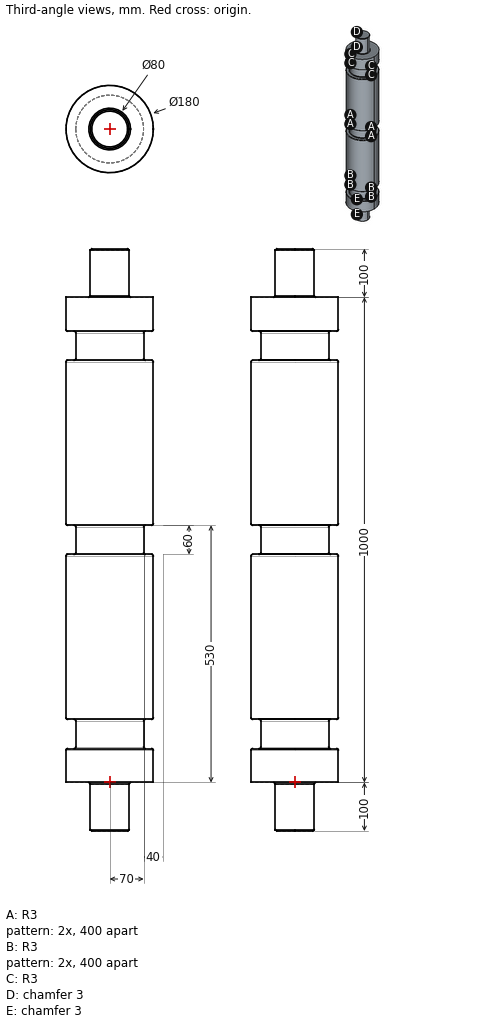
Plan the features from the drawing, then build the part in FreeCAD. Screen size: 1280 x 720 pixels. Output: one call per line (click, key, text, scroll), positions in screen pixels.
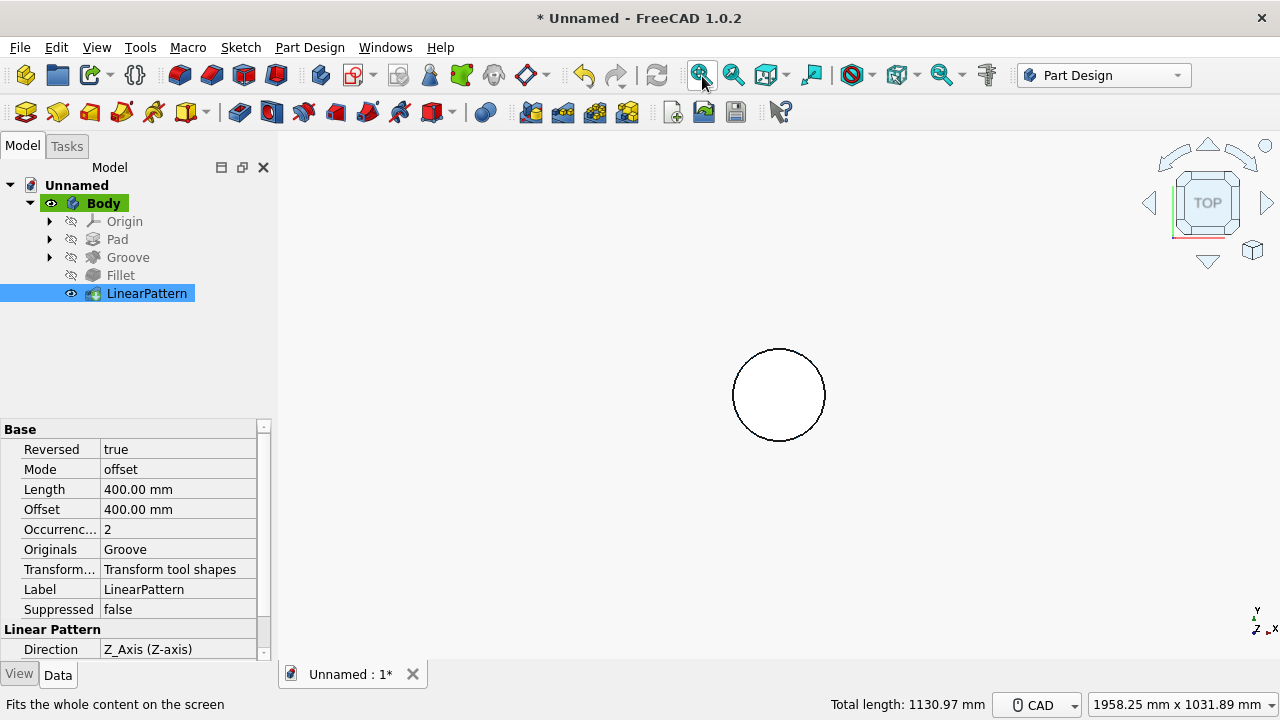
key(0)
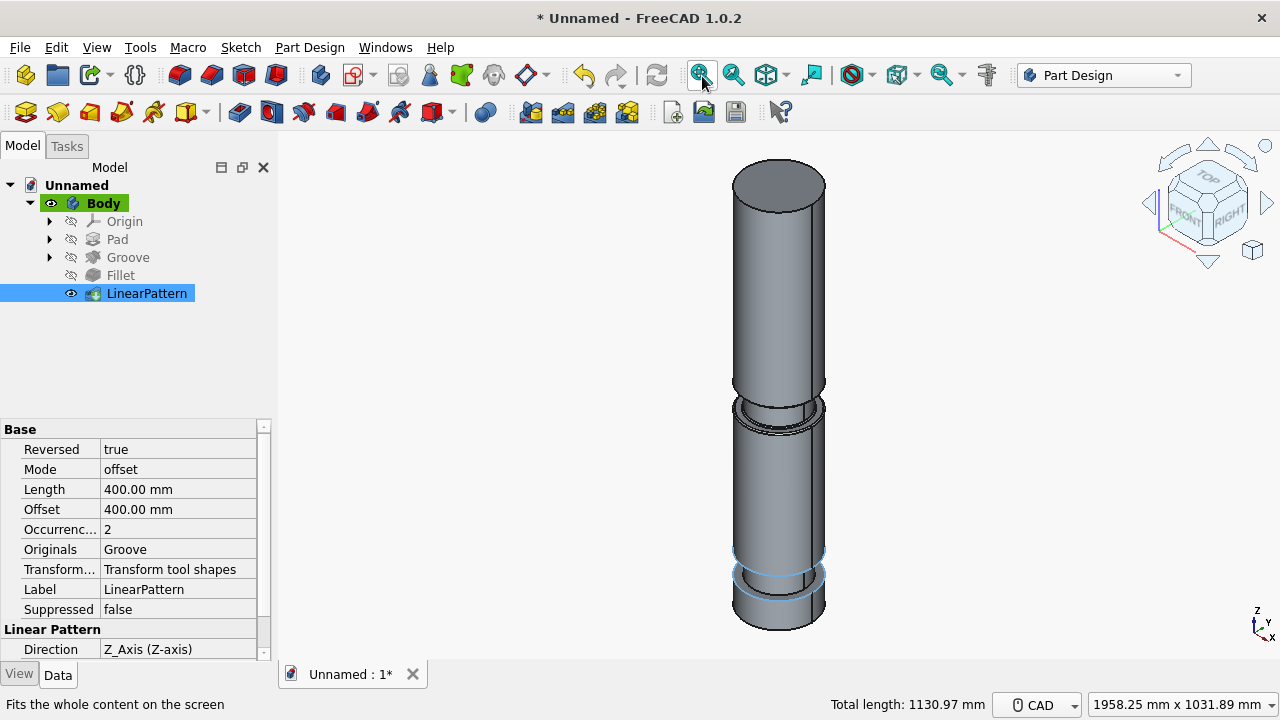
key(1)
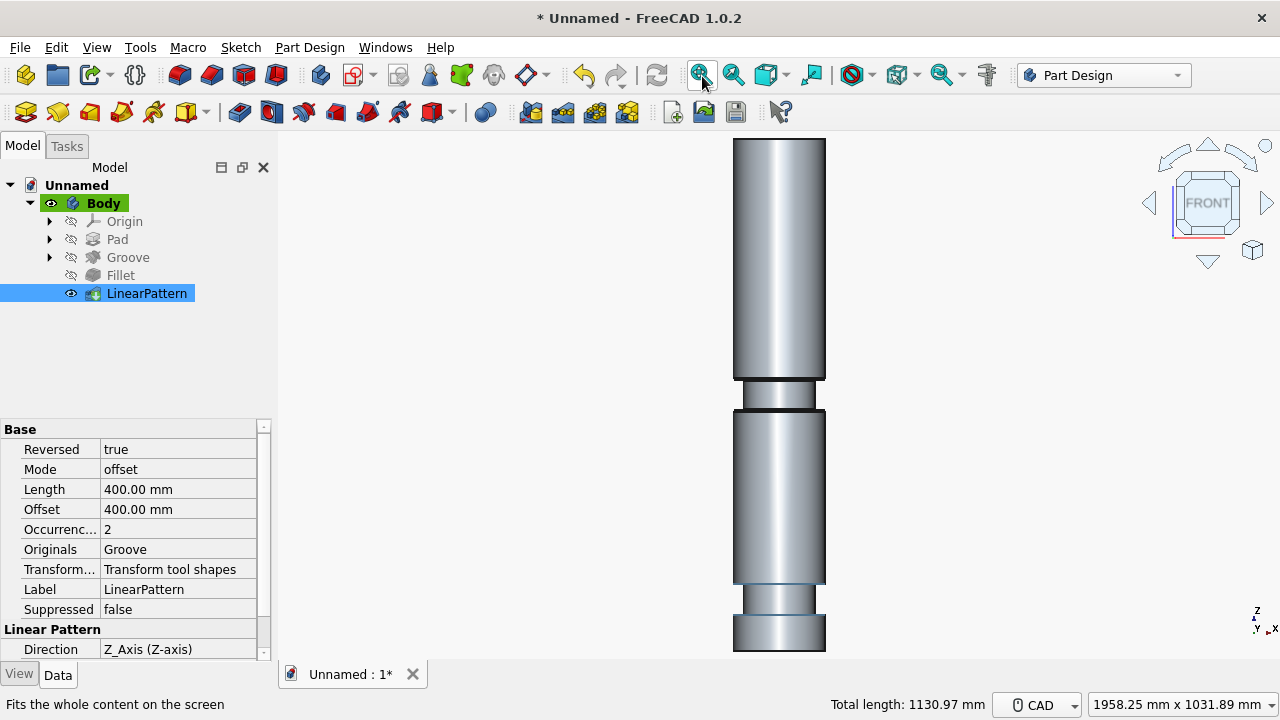
key(3)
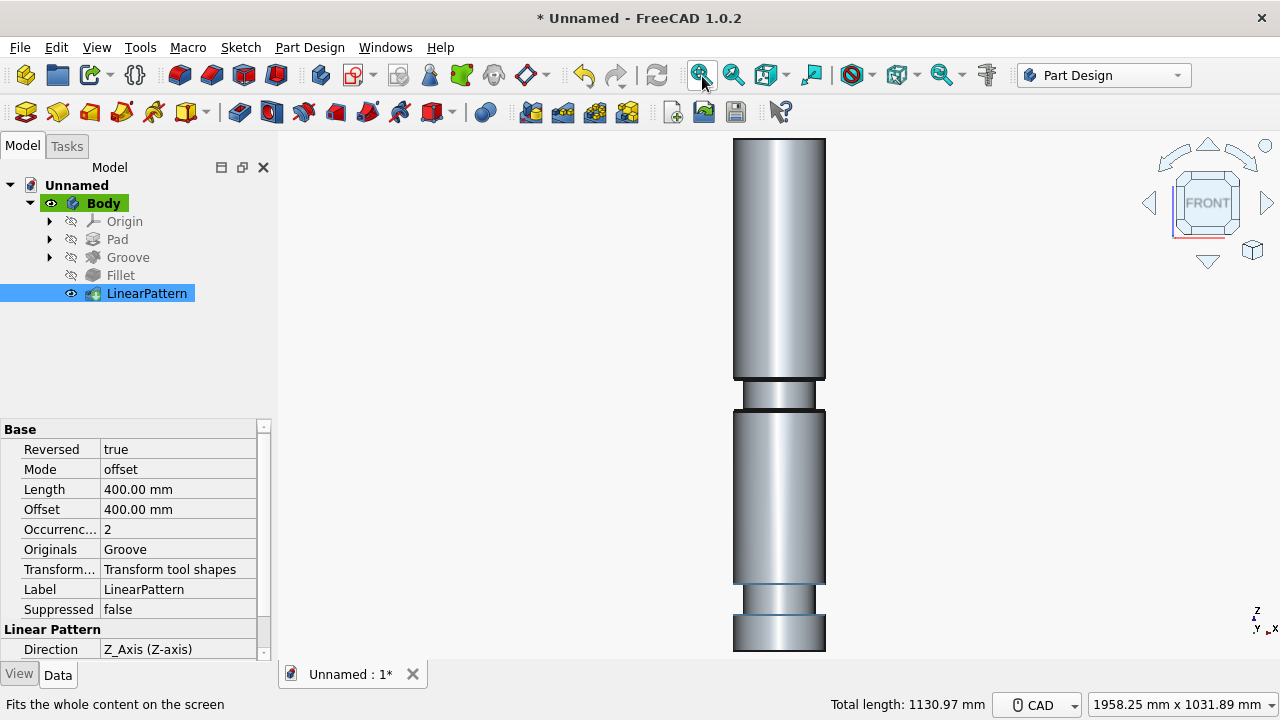
key(5)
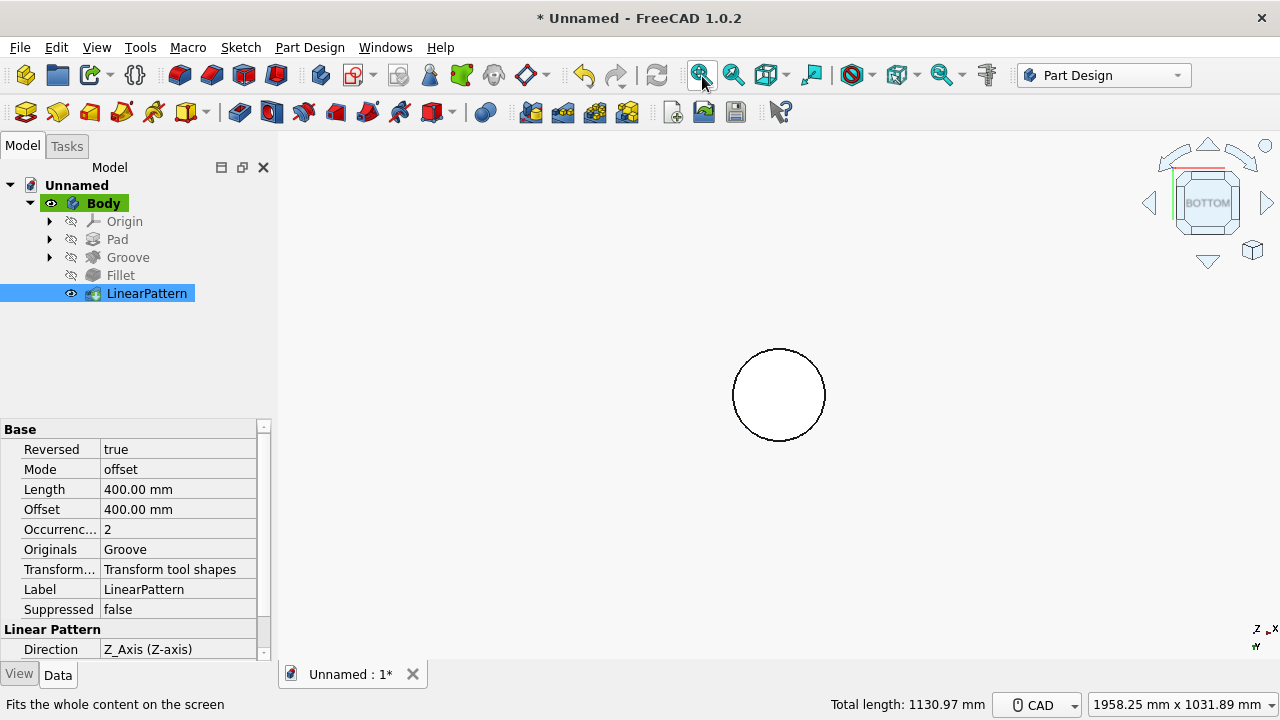
click(702, 76)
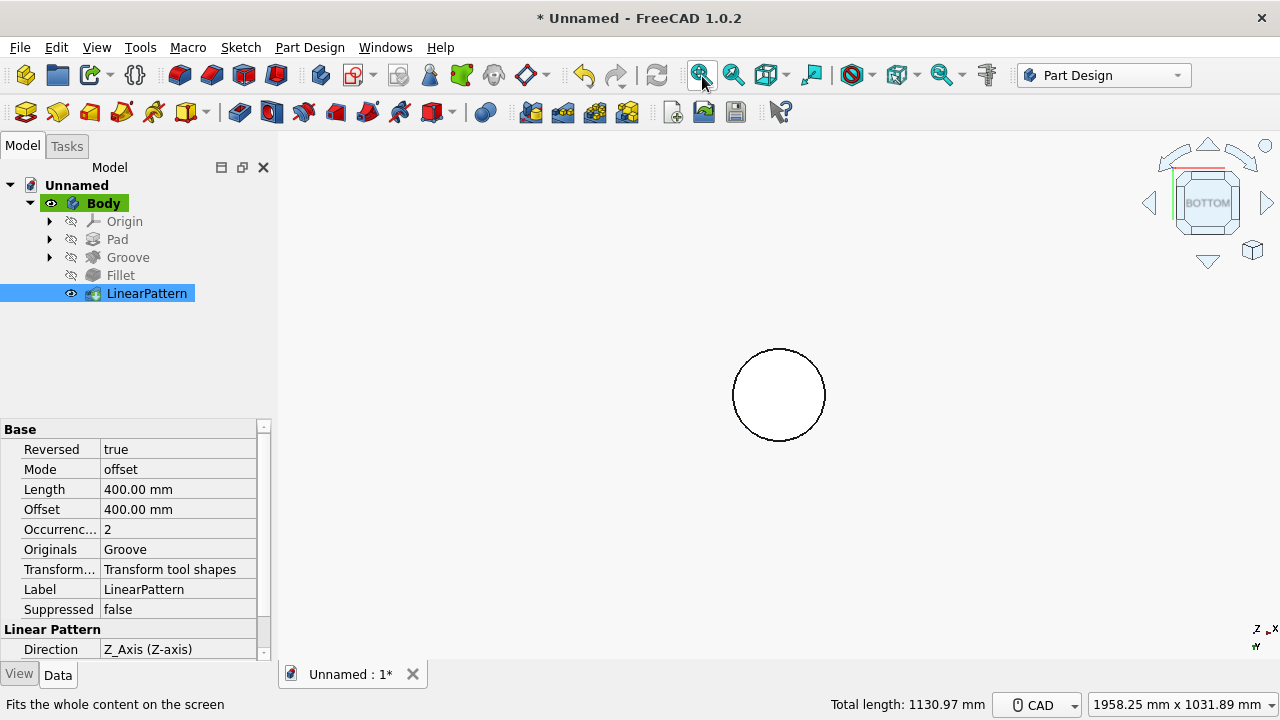
key(4)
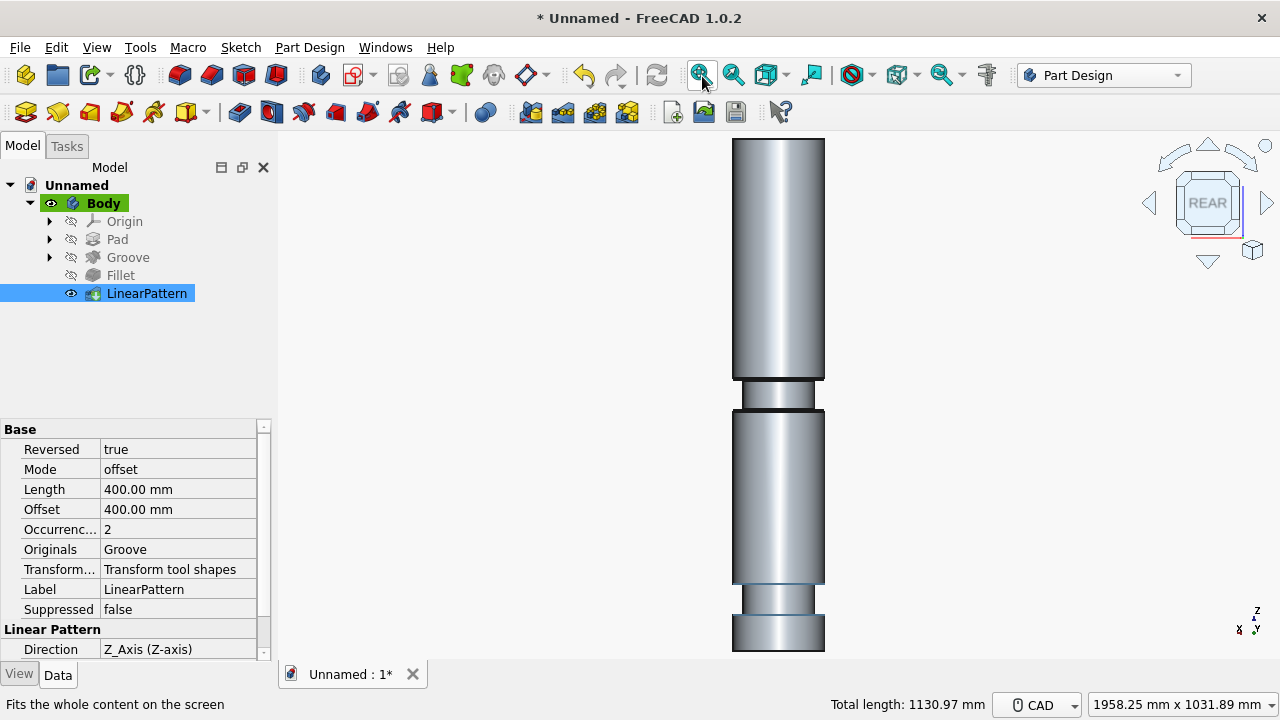
key(6)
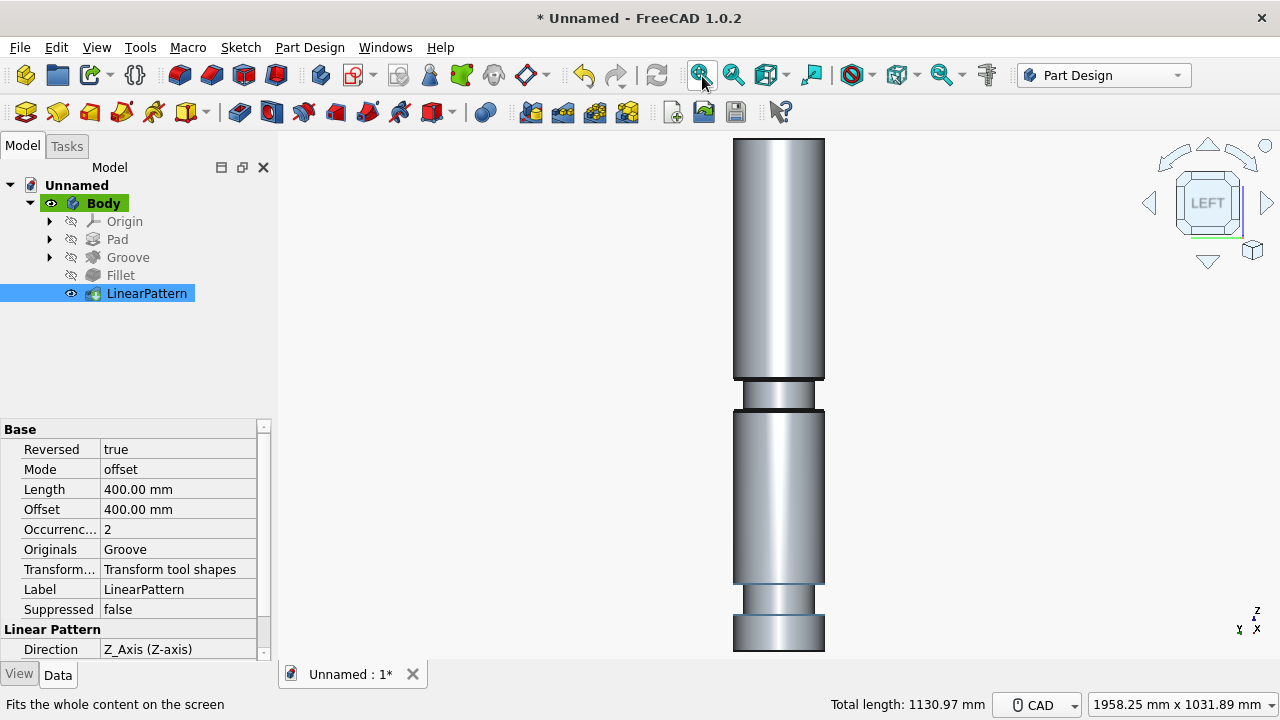
key(v)
key(3)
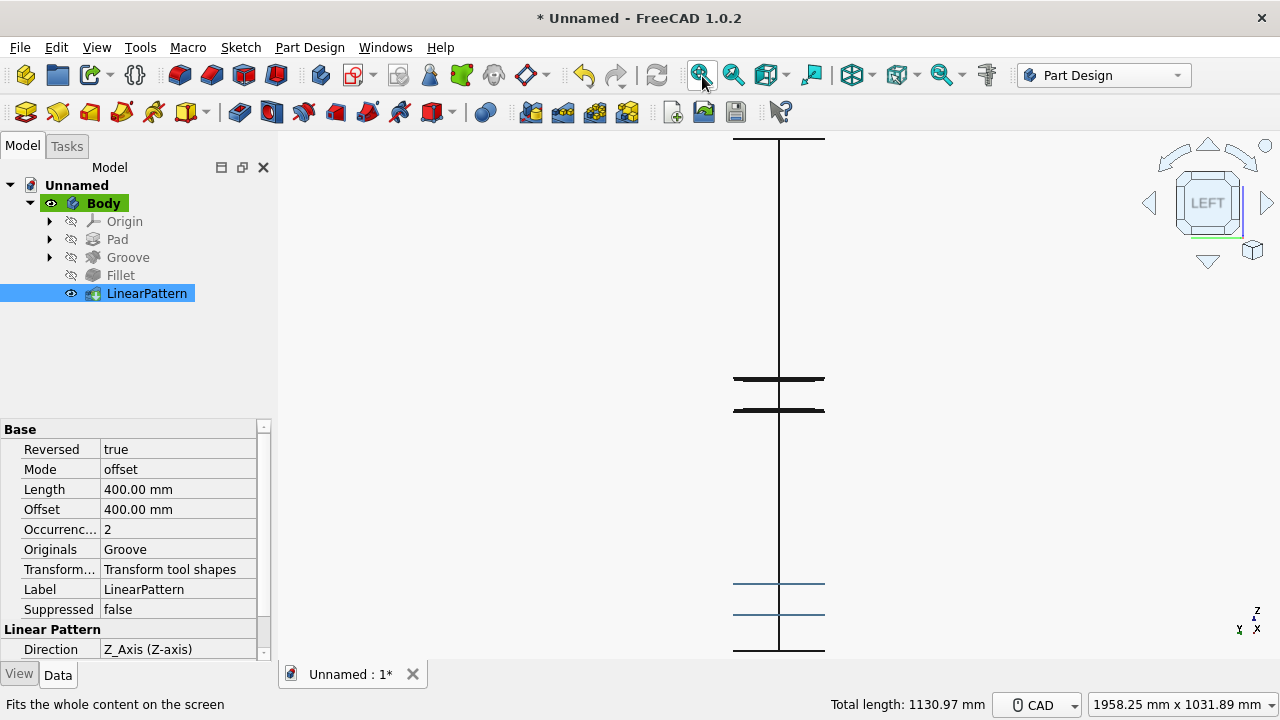
key(0)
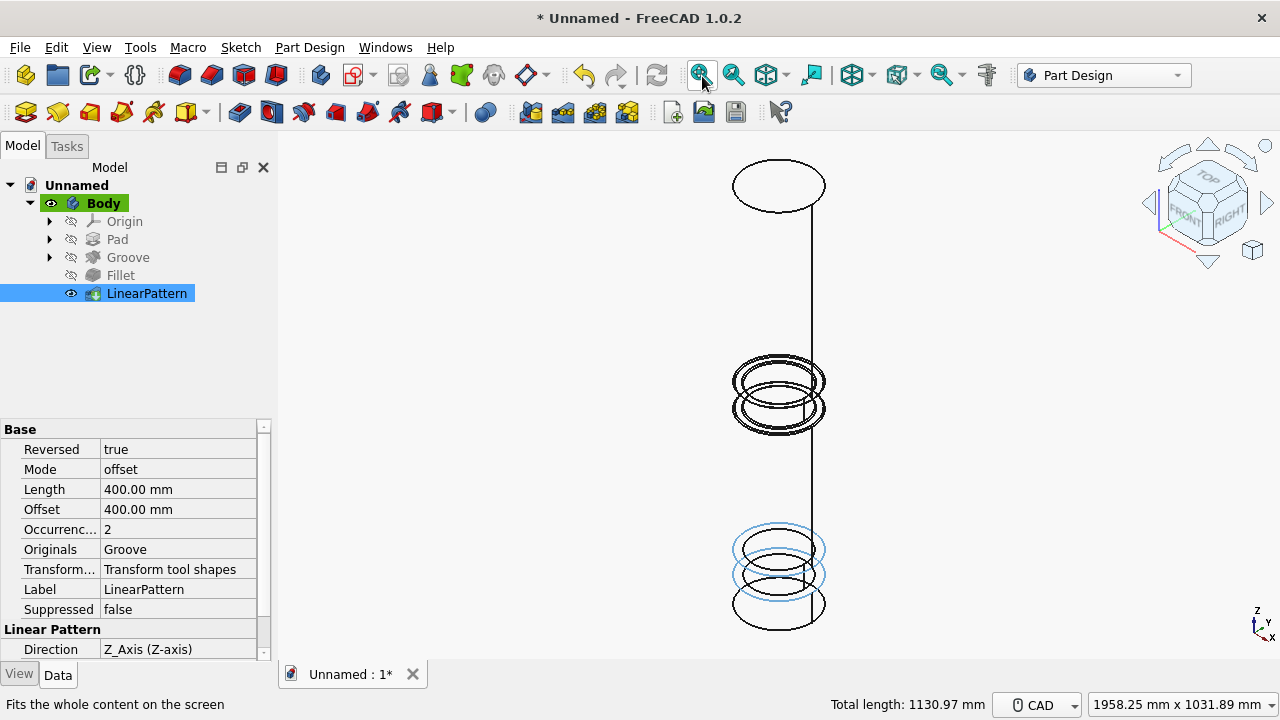
click(754, 534, ctrl)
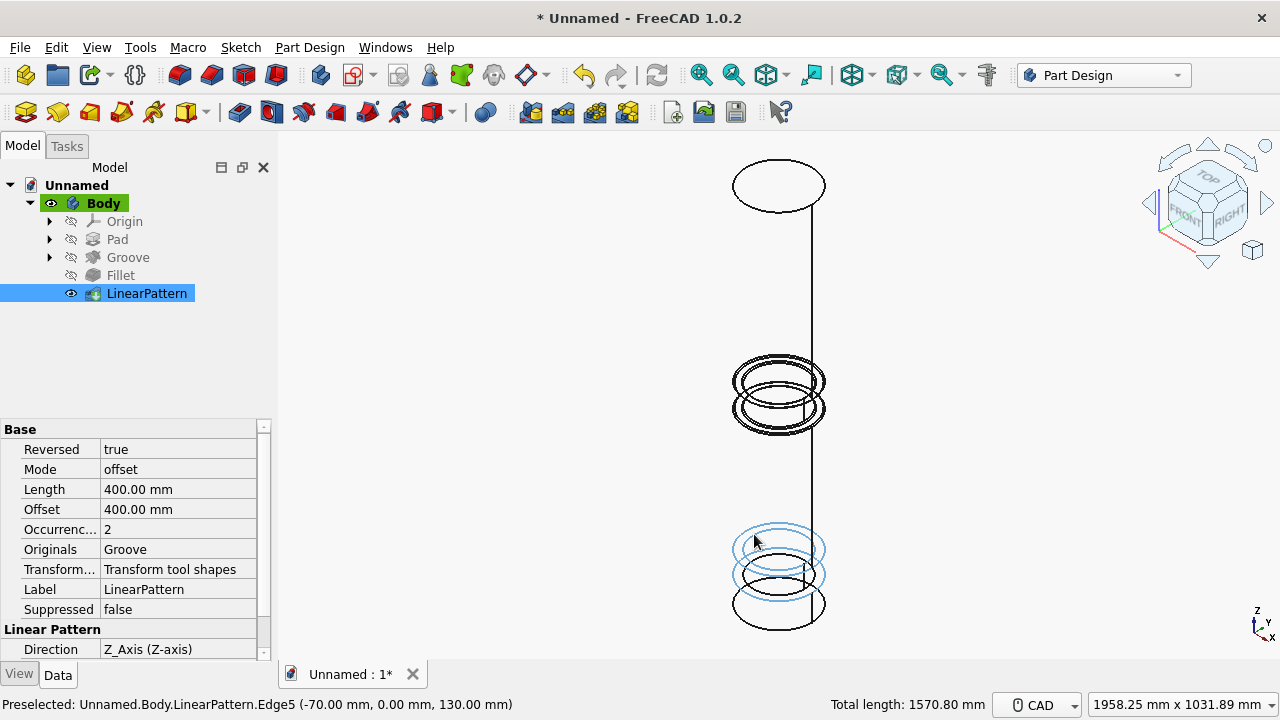
click(773, 553, ctrl)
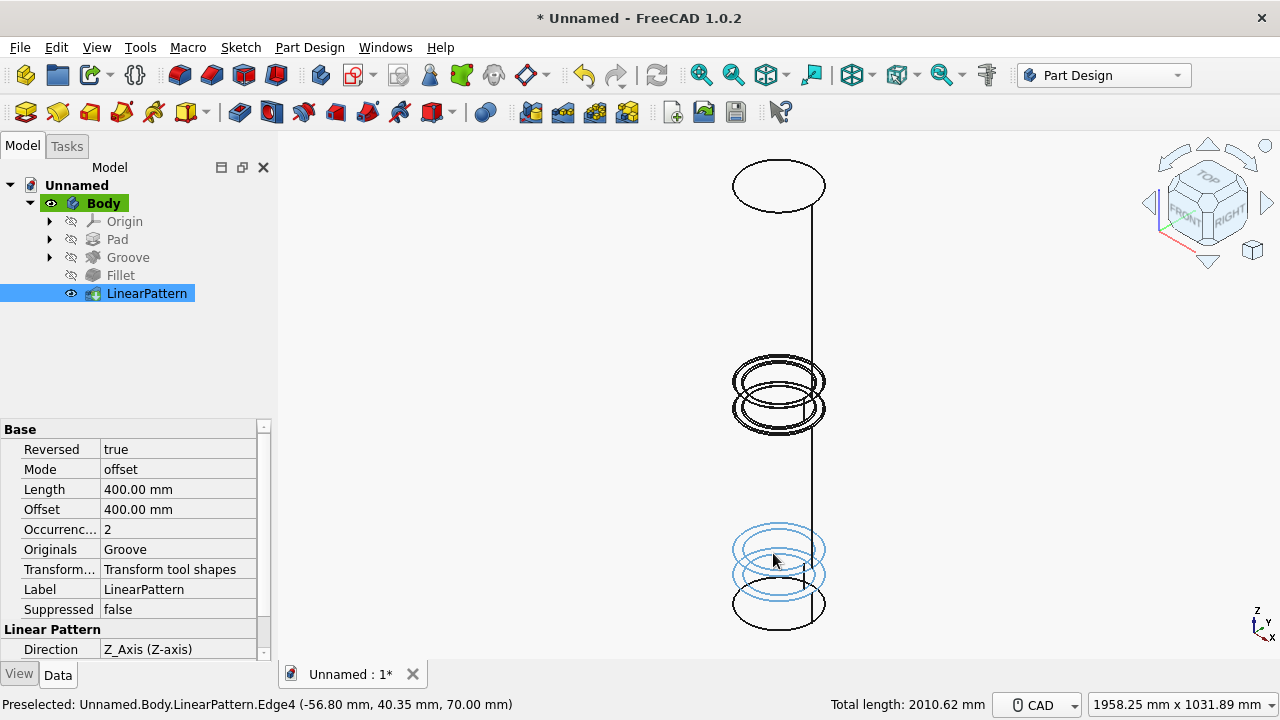
key(v)
key(1)